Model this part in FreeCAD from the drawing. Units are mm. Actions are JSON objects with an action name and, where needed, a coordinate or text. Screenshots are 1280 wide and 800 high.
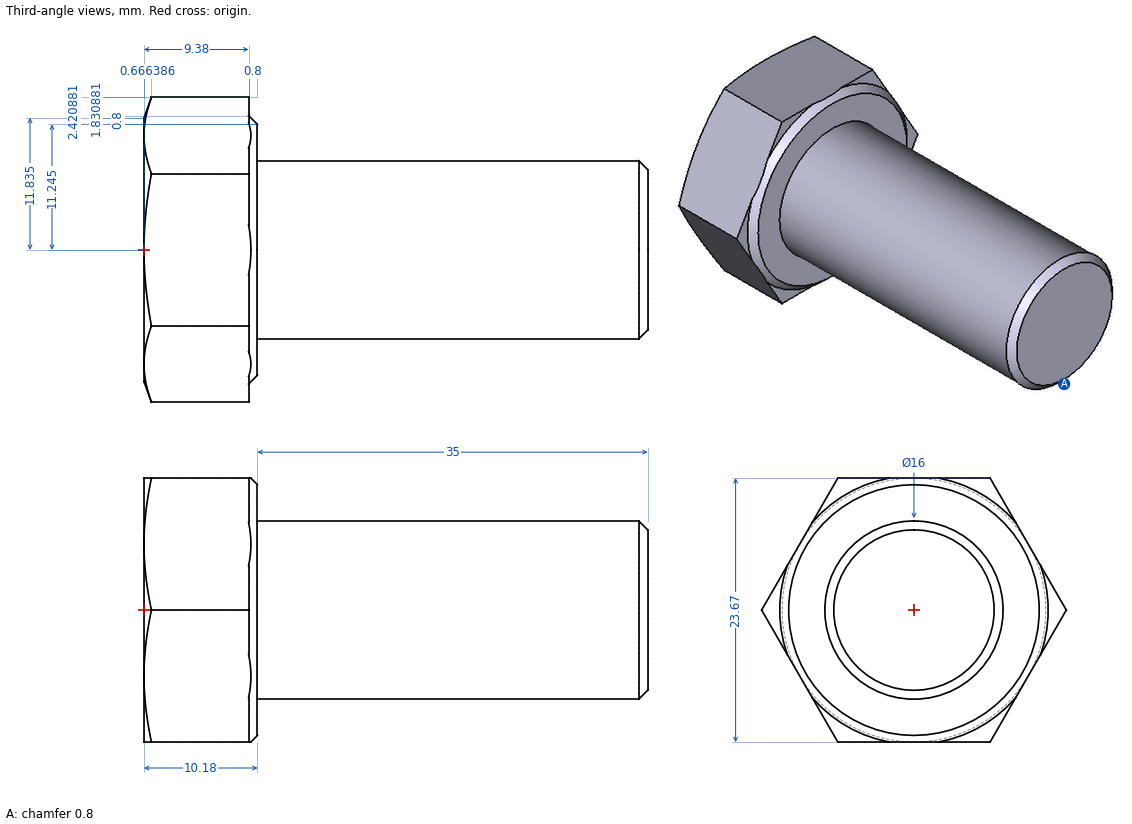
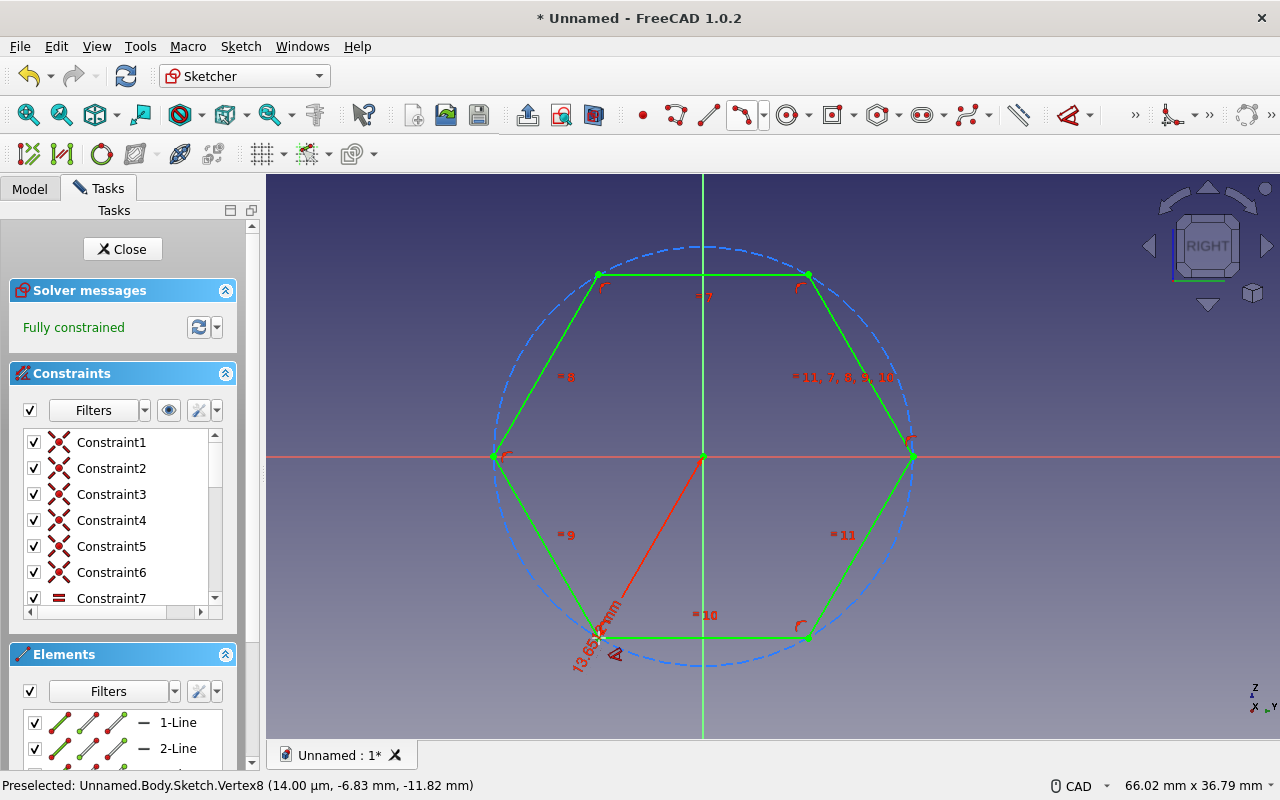
{"action": "left_click", "coordinate": [808, 275]}
{"action": "left_click", "coordinate": [842, 373]}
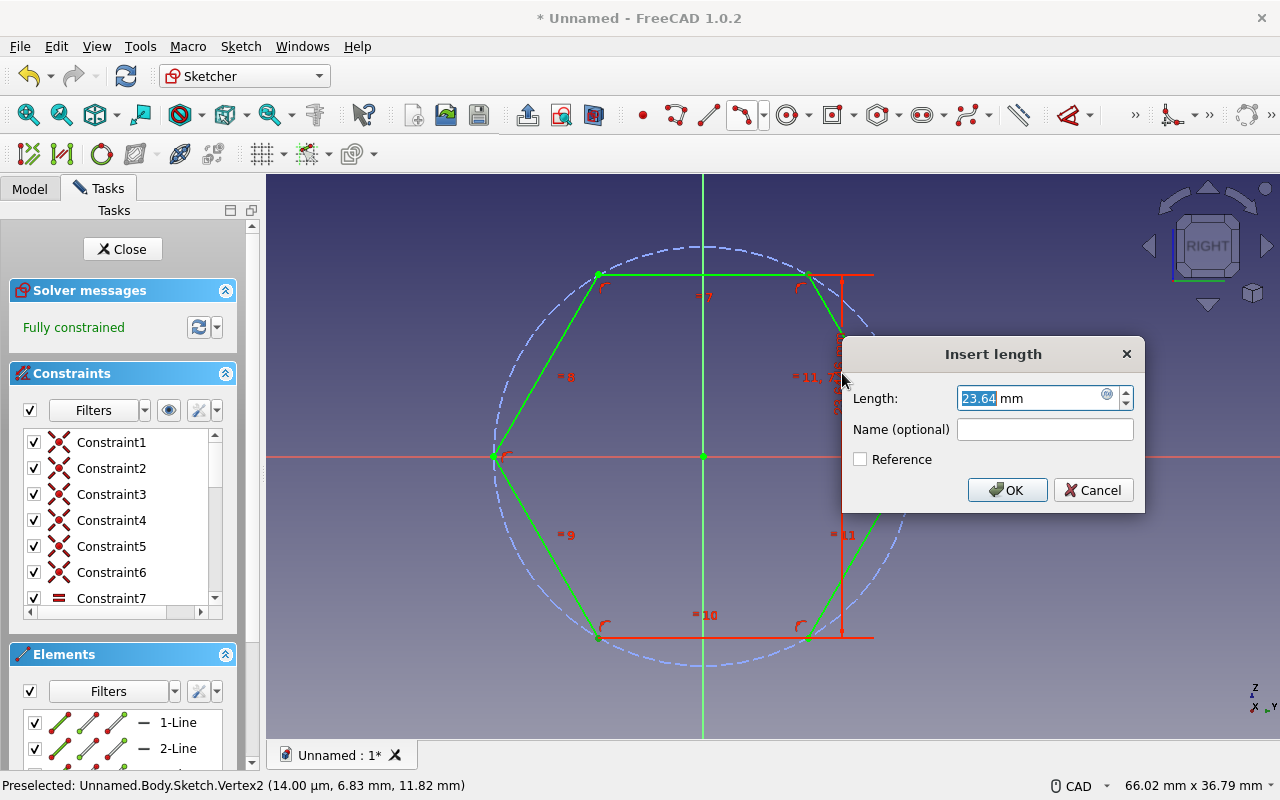
{"action": "type", "text": "23.67"}
{"action": "key", "text": "Return"}
{"action": "key", "text": "Escape"}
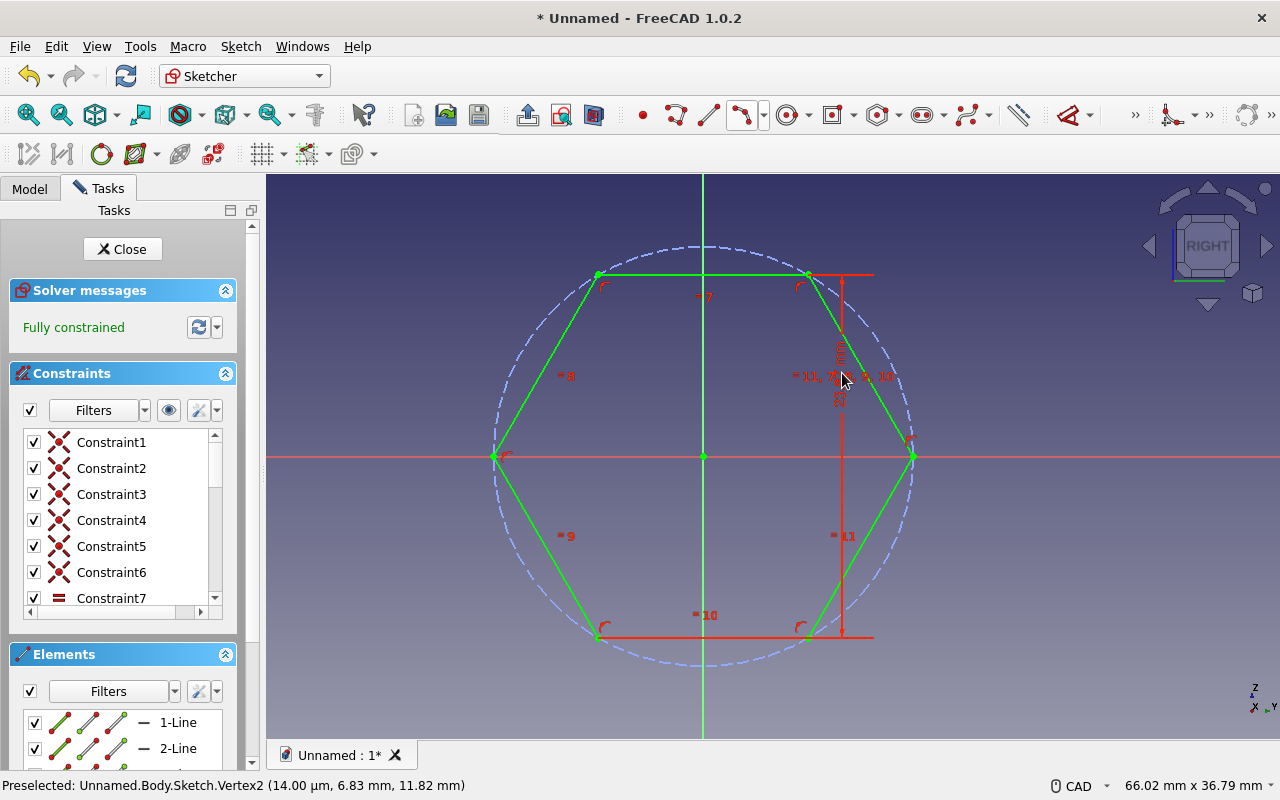
{"action": "left_click", "coordinate": [123, 249]}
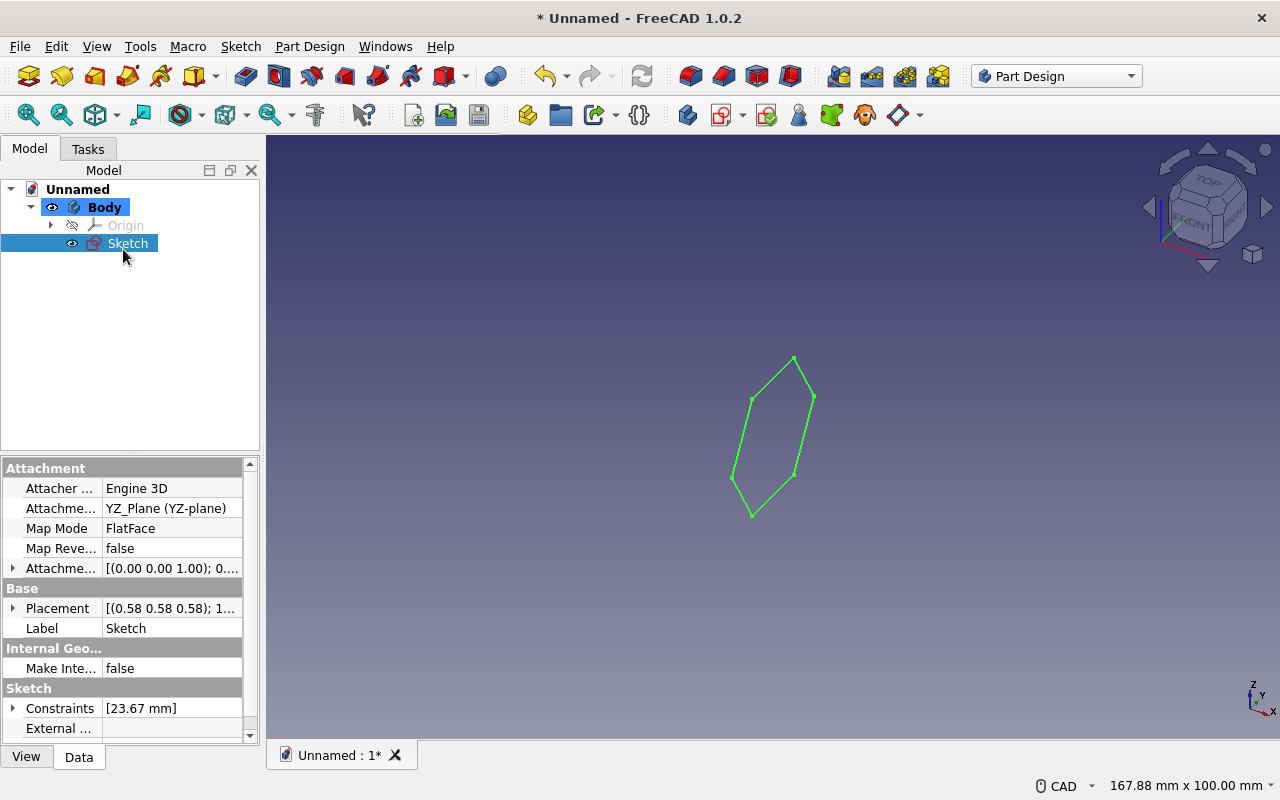
{"action": "left_click", "coordinate": [29, 76]}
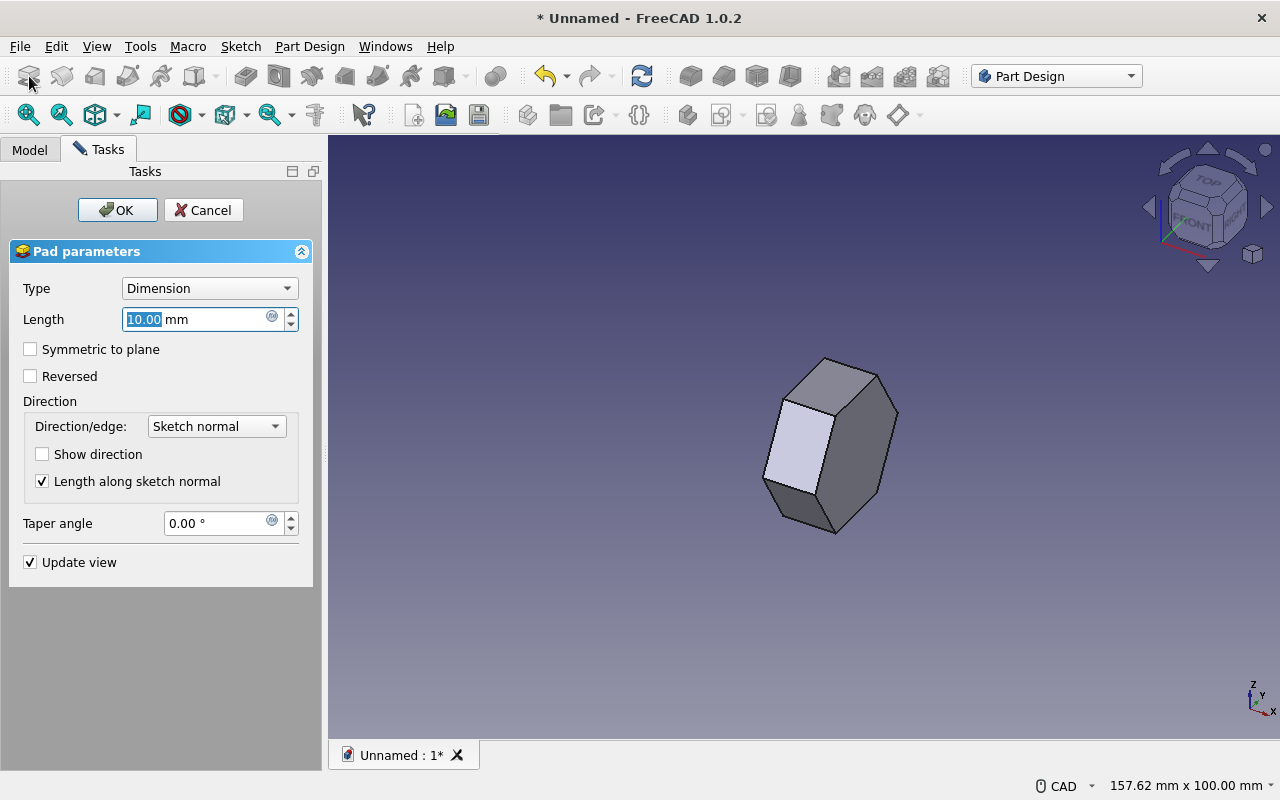
{"action": "type", "text": "10.18"}
{"action": "key", "text": "Tab"}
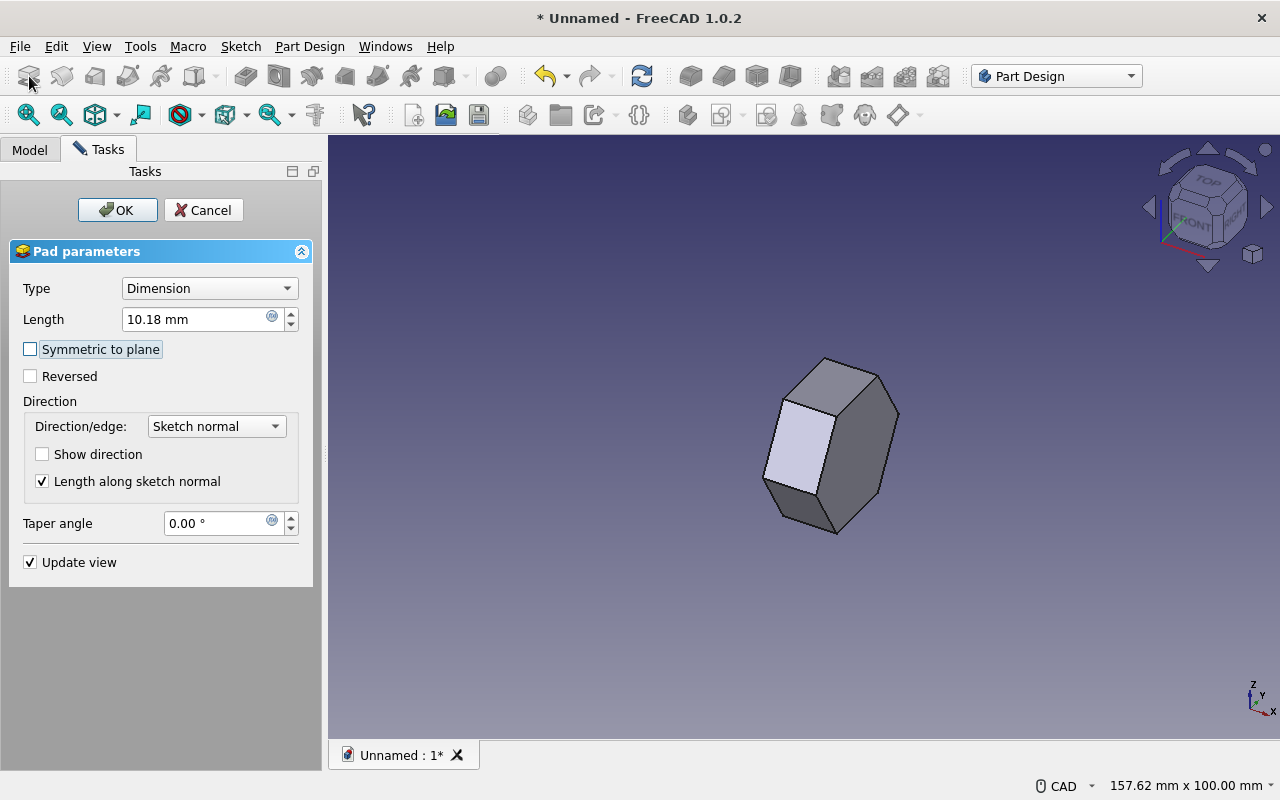
{"action": "left_click", "coordinate": [118, 210]}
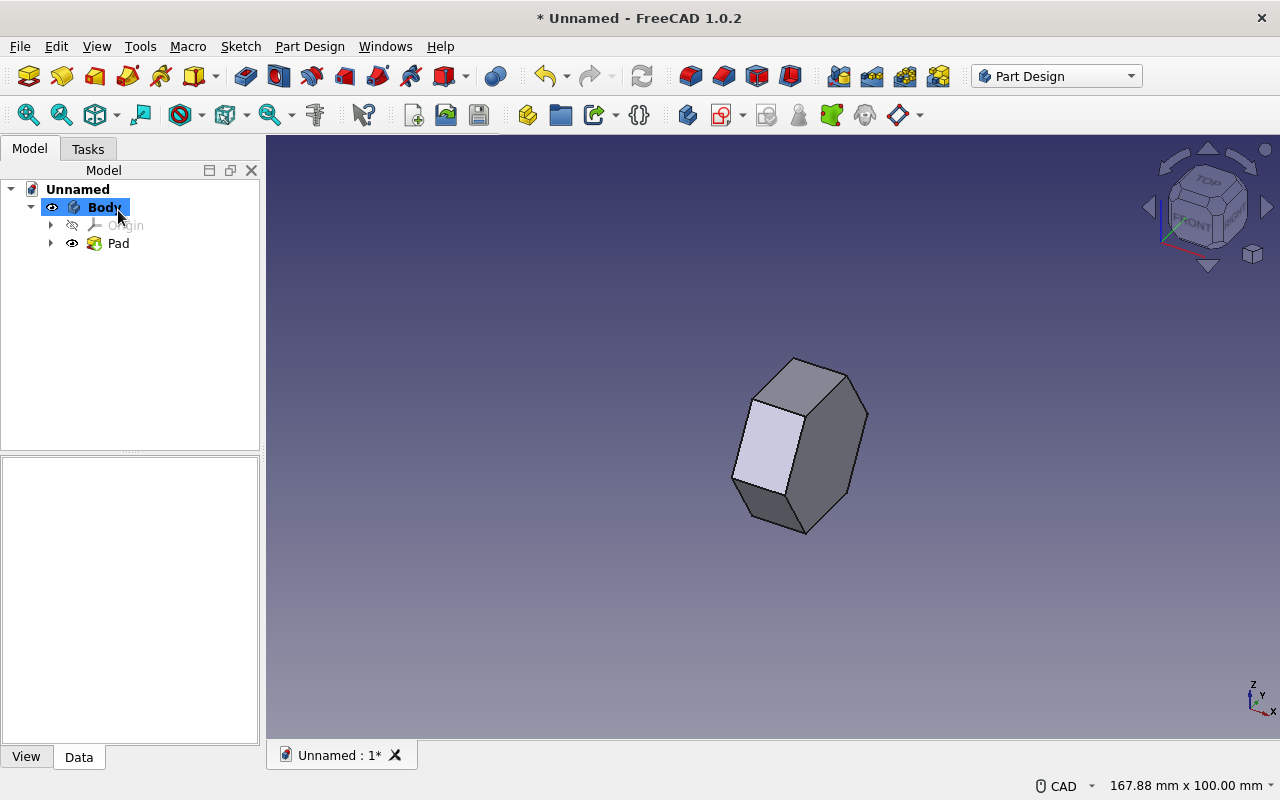
{"action": "key", "text": "v f"}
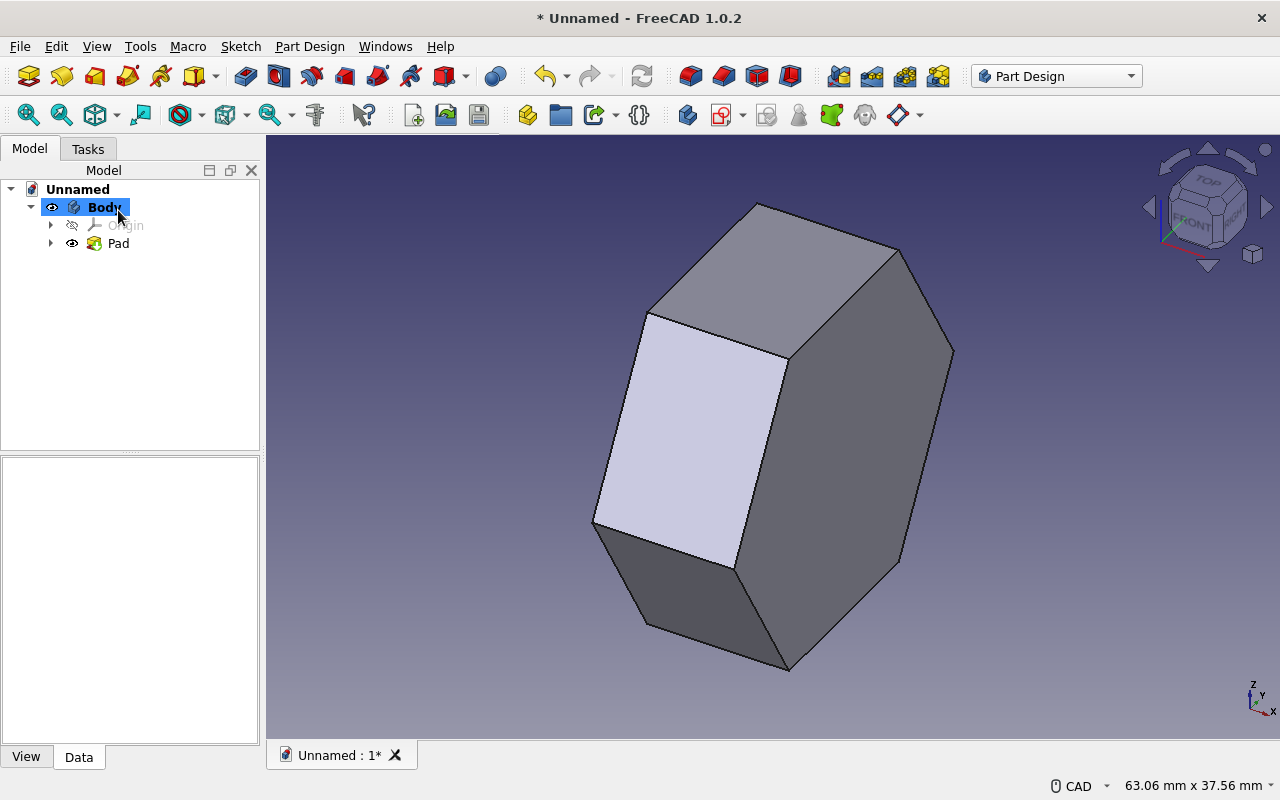
{"action": "left_click", "coordinate": [720, 116]}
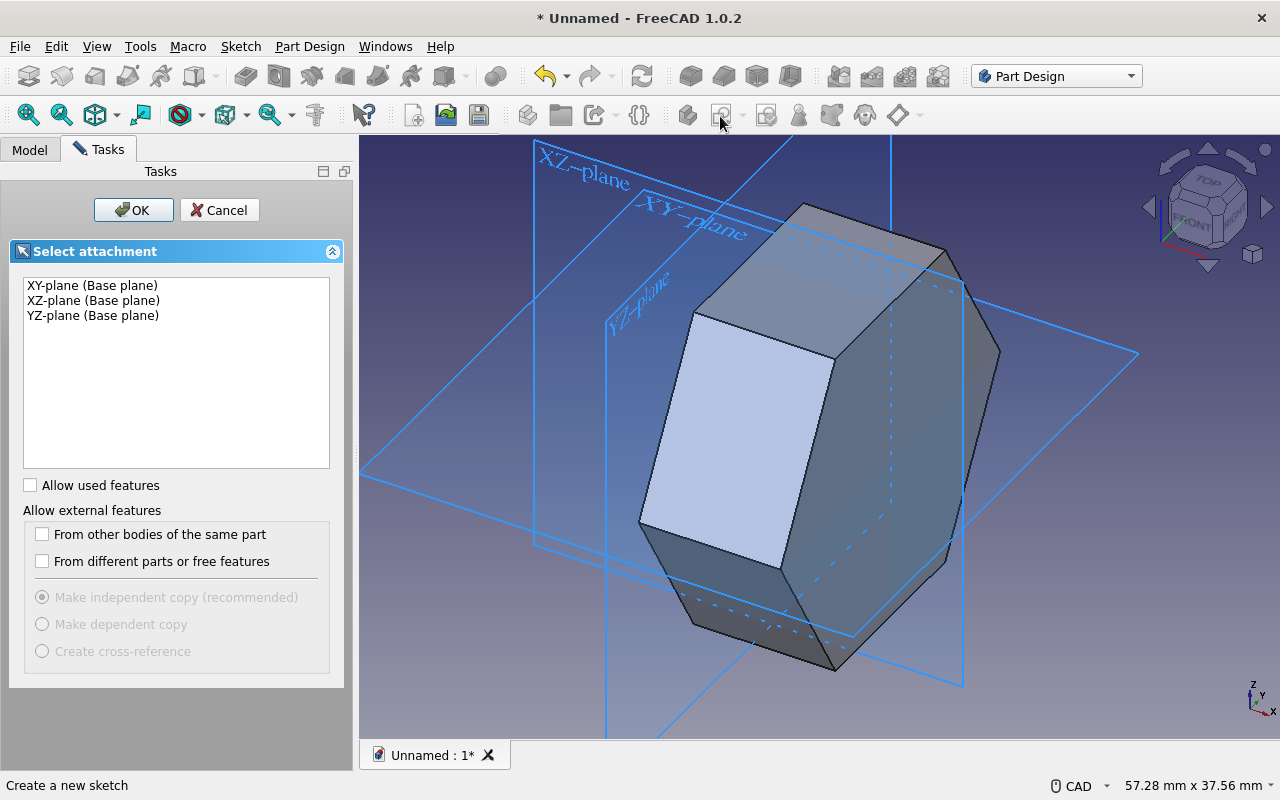
{"action": "left_click", "coordinate": [84, 286]}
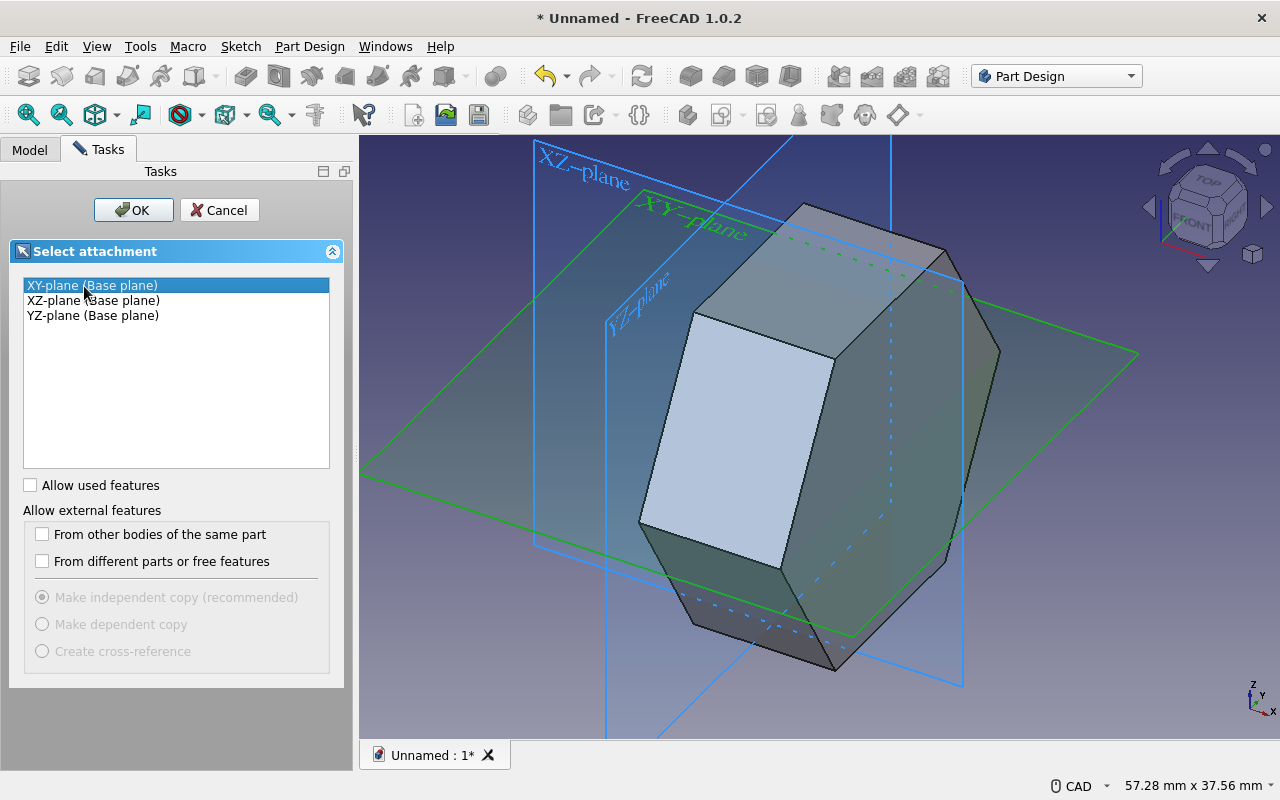
{"action": "left_click", "coordinate": [134, 210]}